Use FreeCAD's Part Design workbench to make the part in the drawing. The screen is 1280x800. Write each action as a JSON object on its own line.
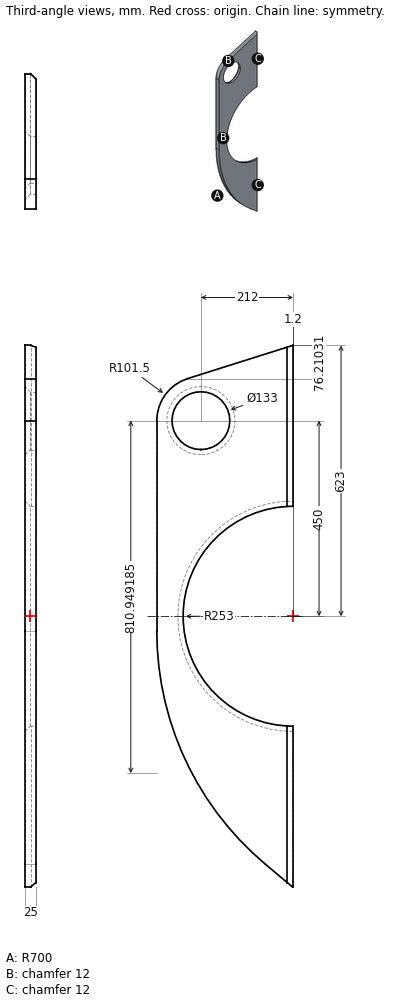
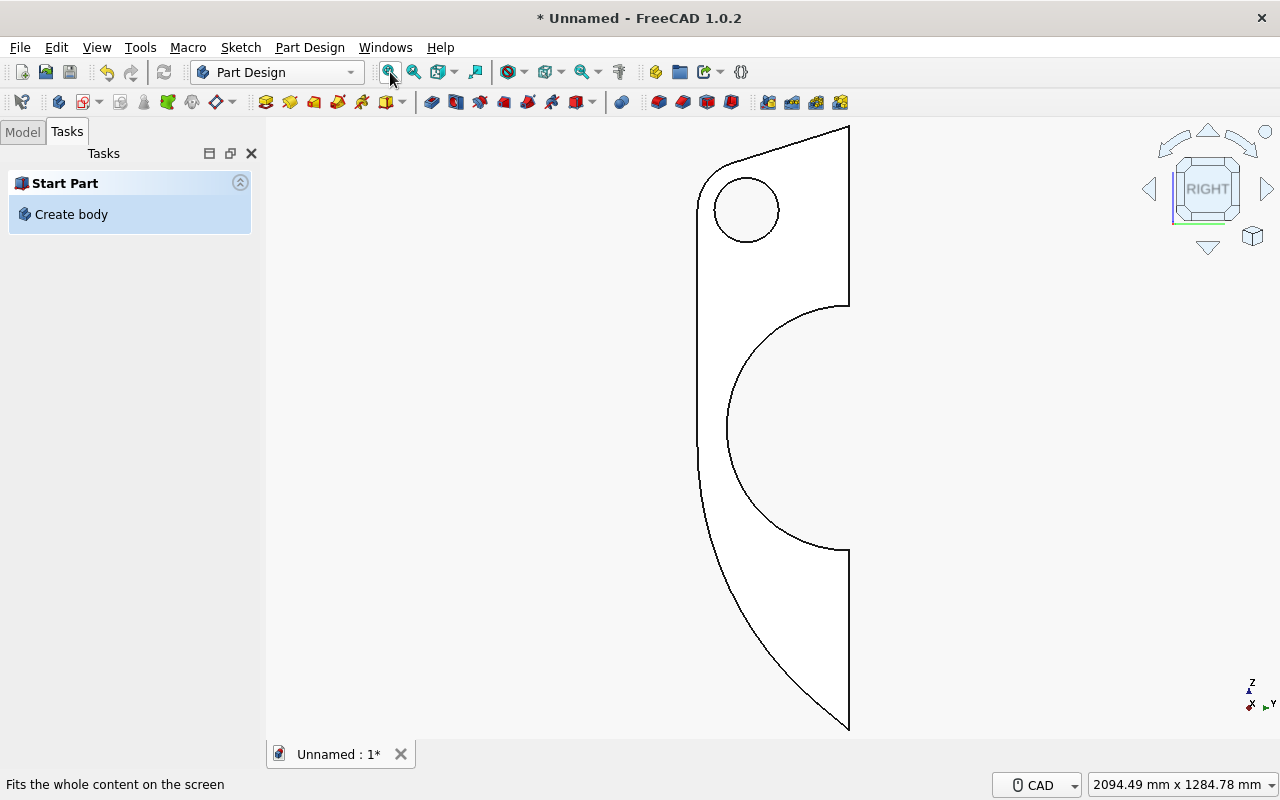
{"action": "left_click", "coordinate": [849, 639]}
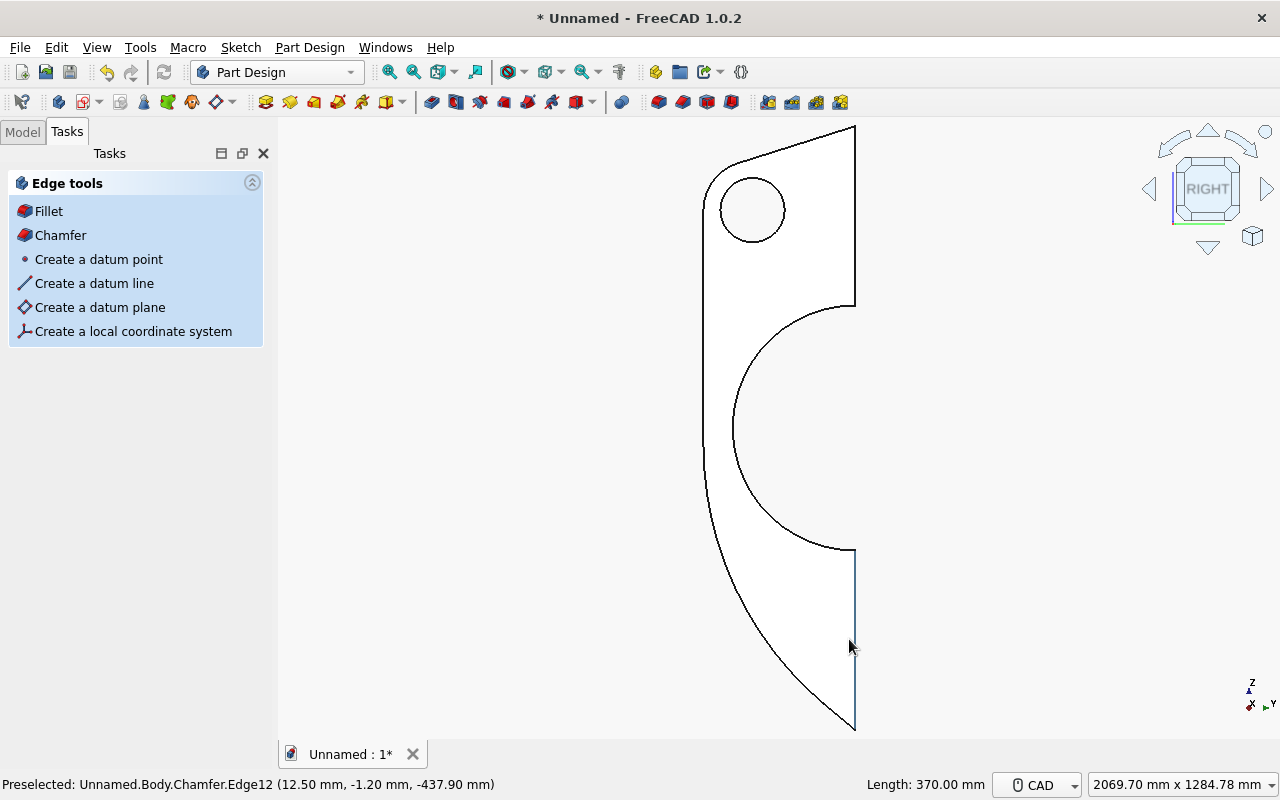
{"action": "left_click", "coordinate": [855, 215], "text": "ctrl"}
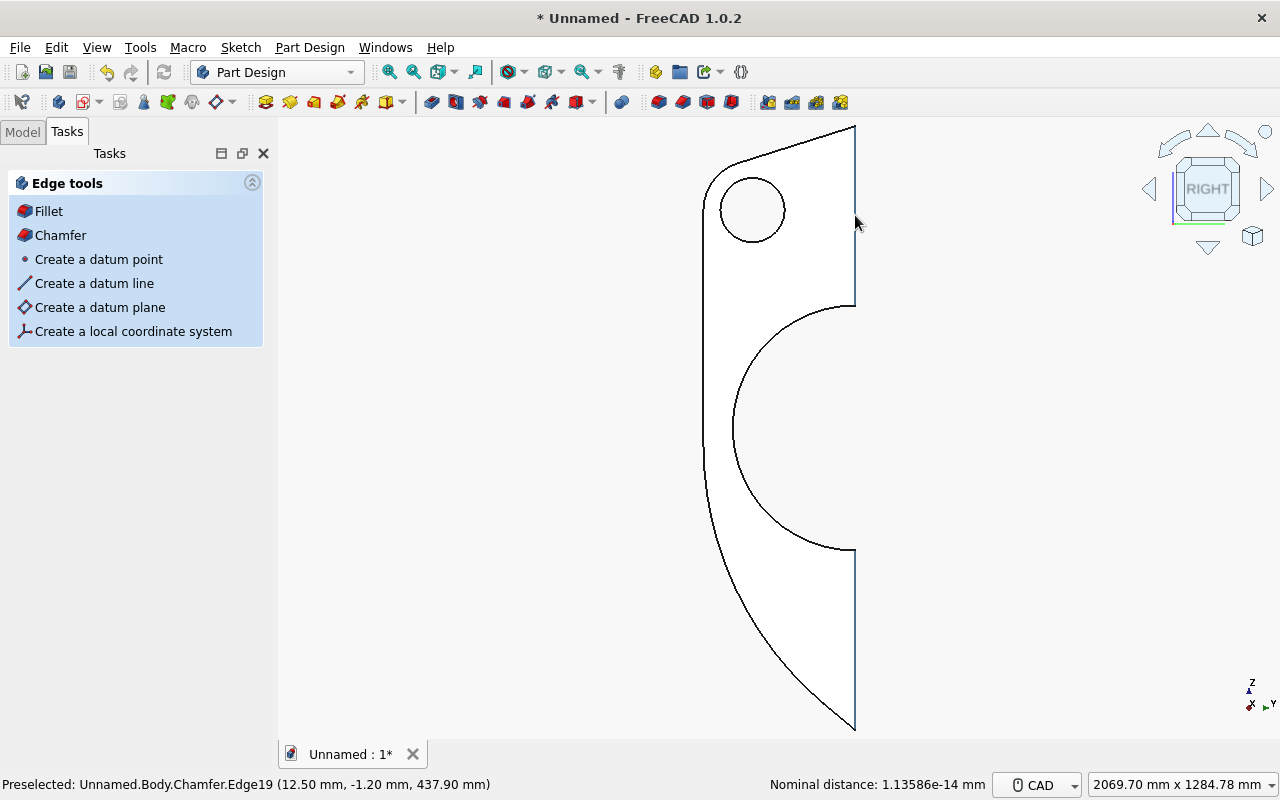
{"action": "left_click", "coordinate": [684, 102]}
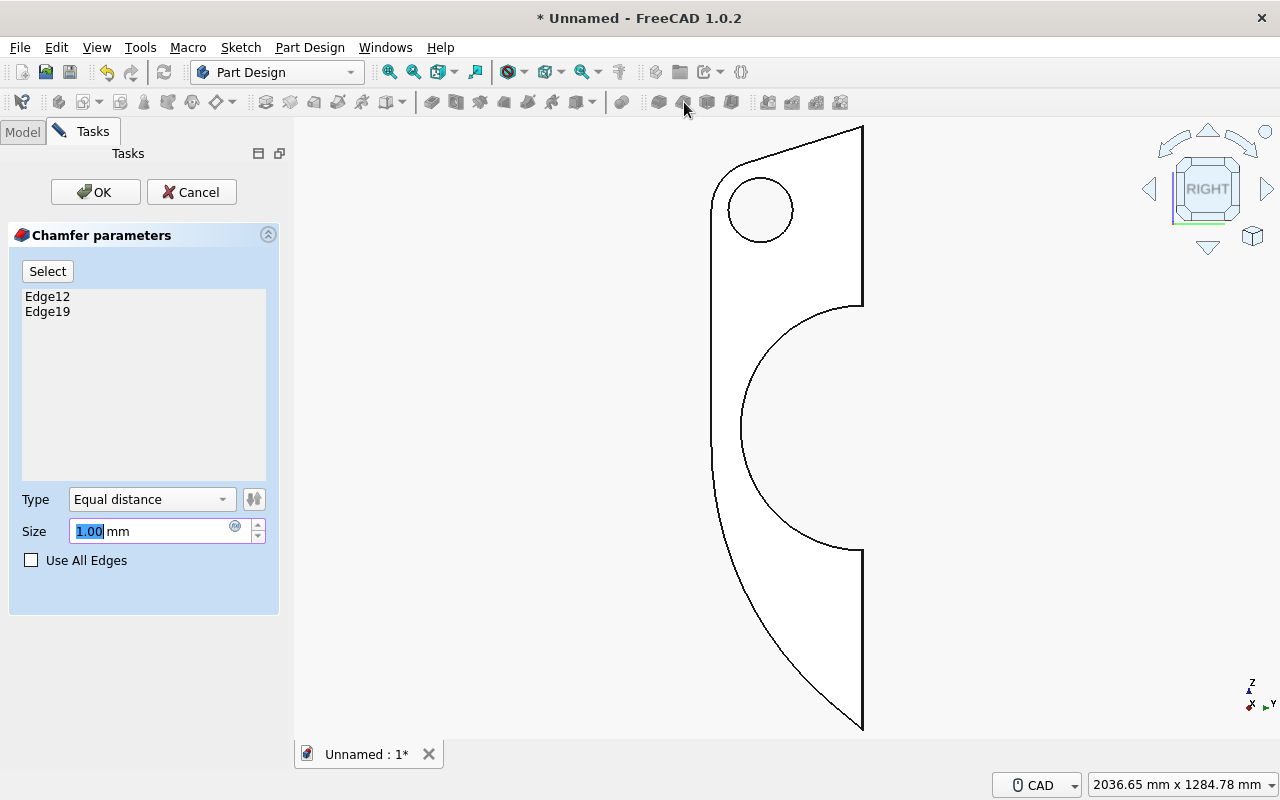
{"action": "type", "text": "12"}
{"action": "key", "text": "Tab"}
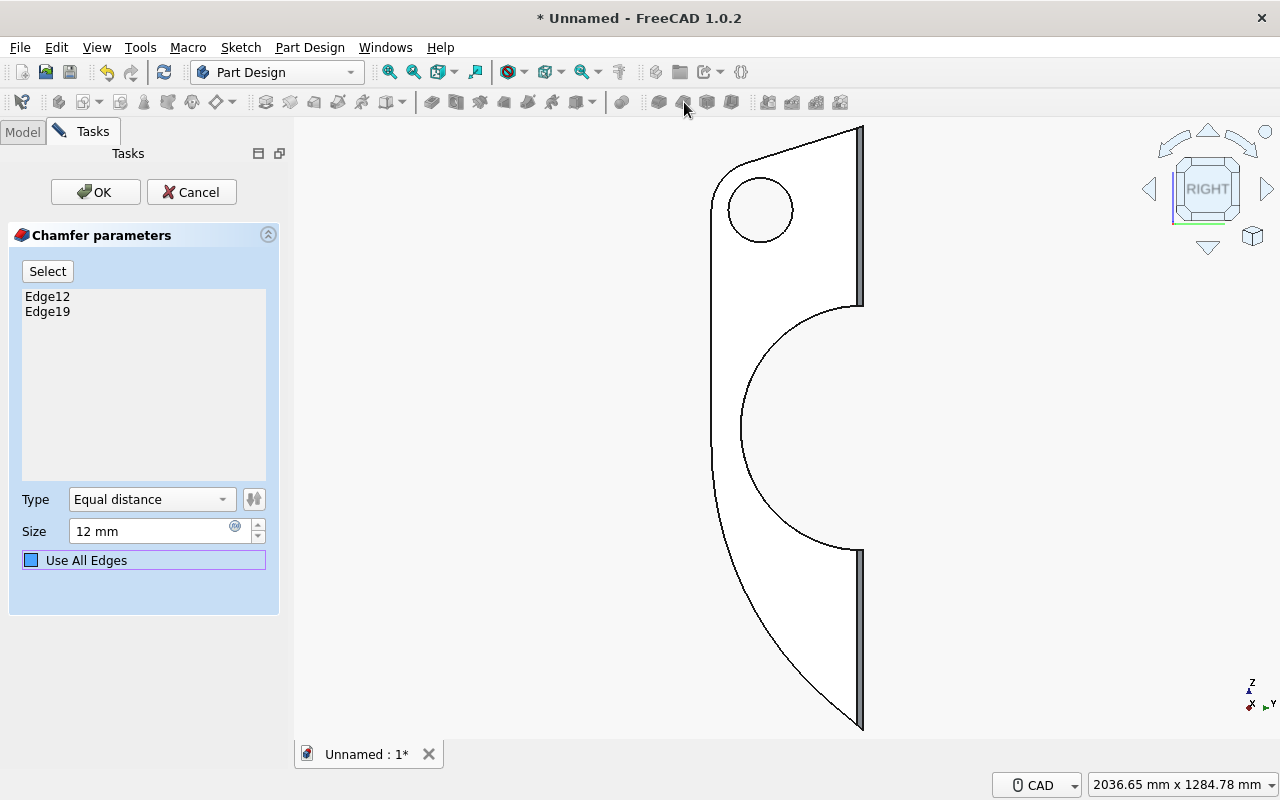
{"action": "left_click", "coordinate": [96, 192]}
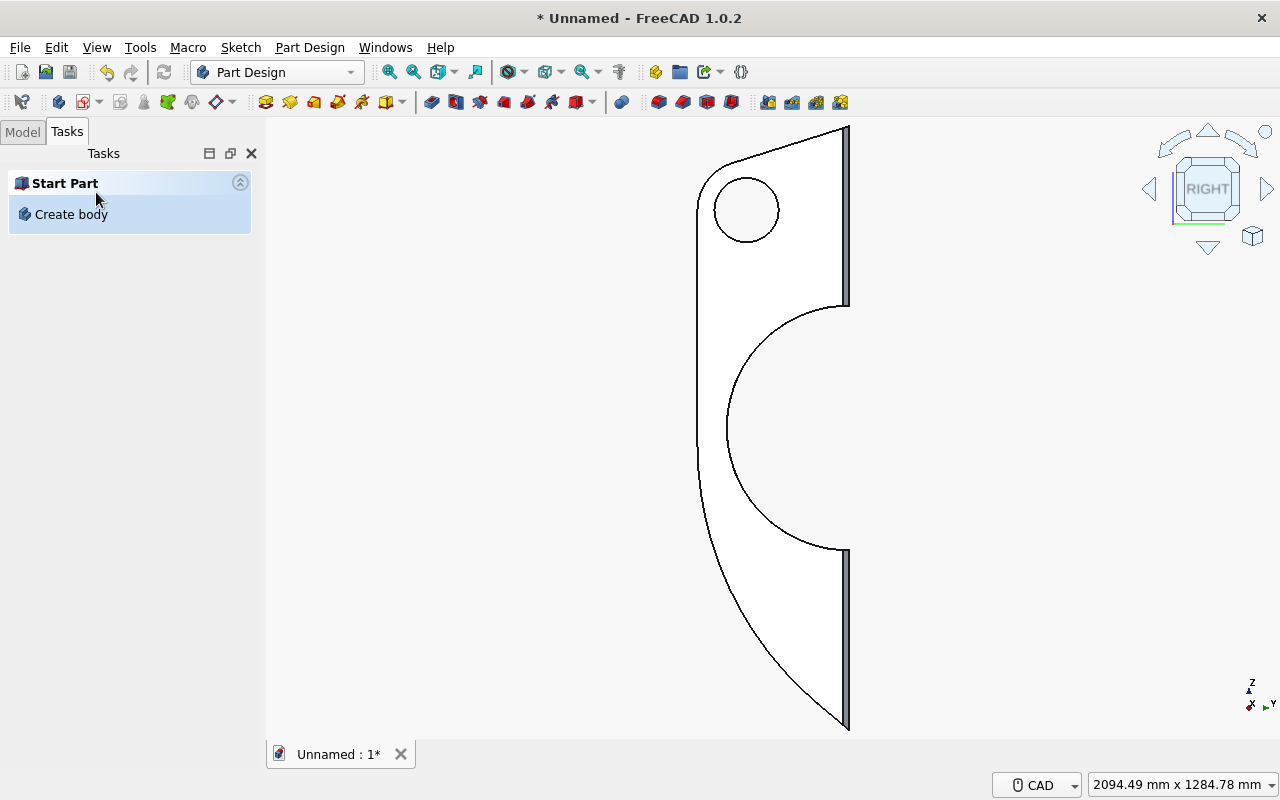
{"action": "key", "text": "0"}